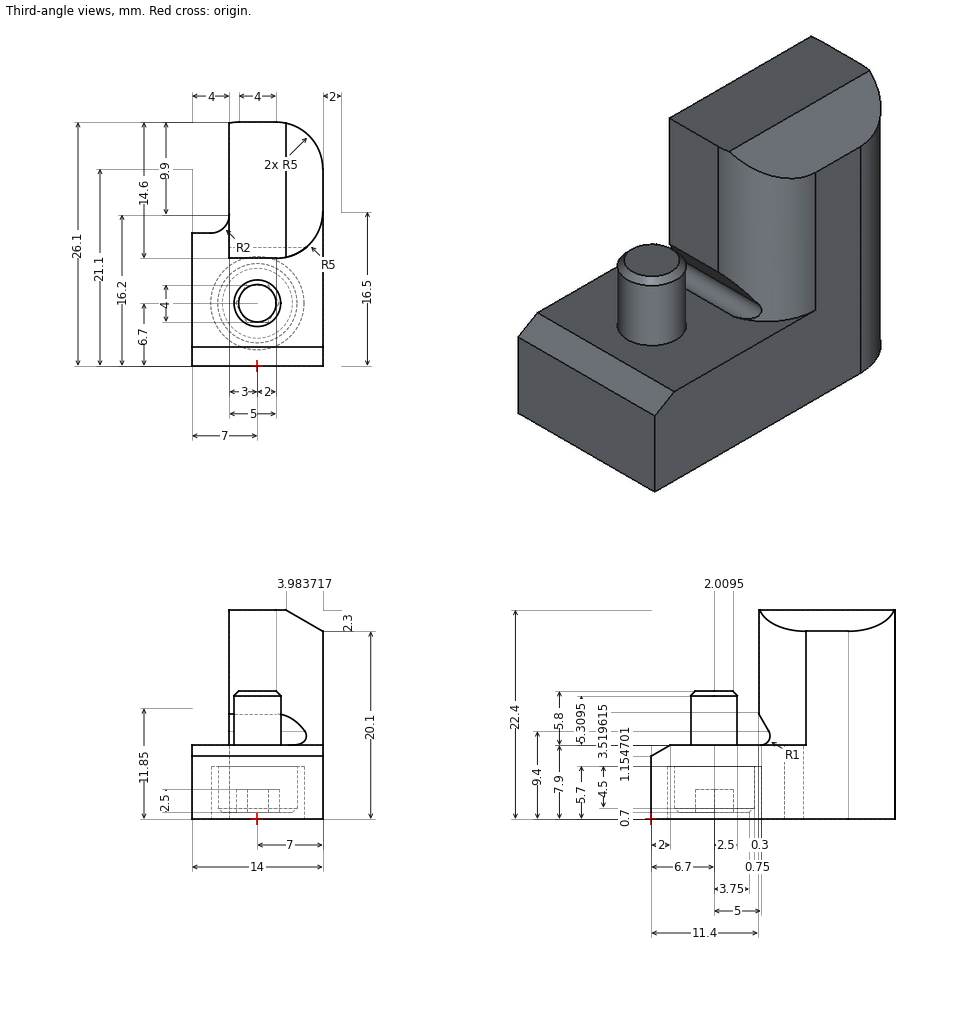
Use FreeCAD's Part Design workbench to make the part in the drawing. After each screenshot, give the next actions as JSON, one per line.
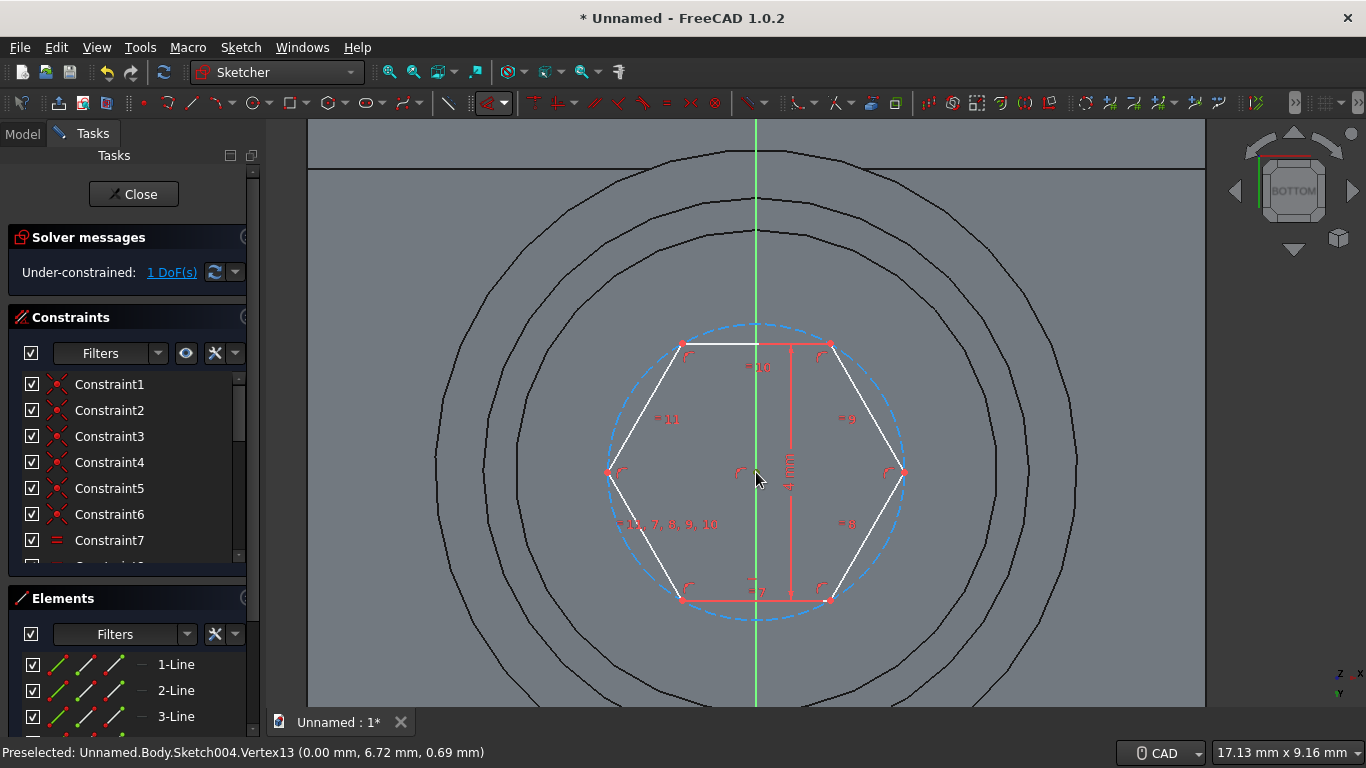
{"action": "left_click", "coordinate": [506, 104]}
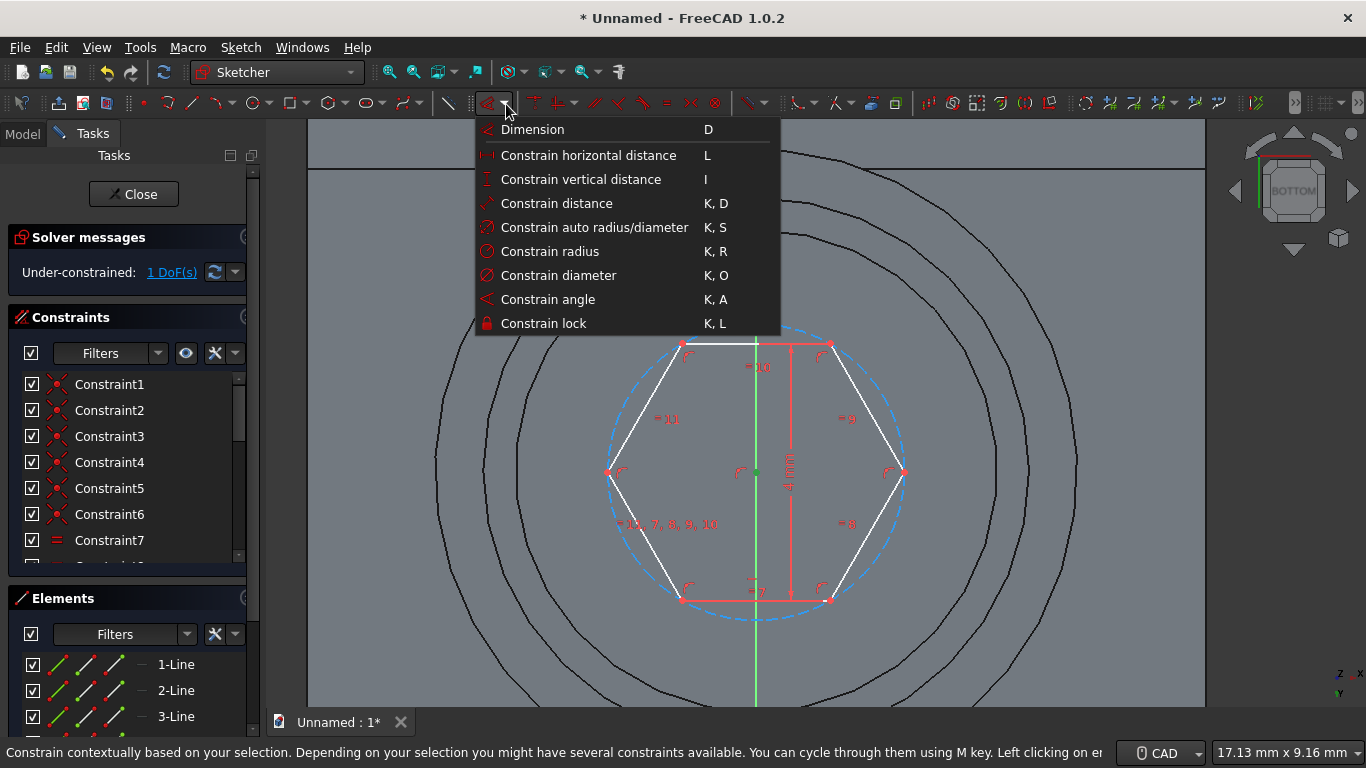
{"action": "left_click", "coordinate": [628, 179]}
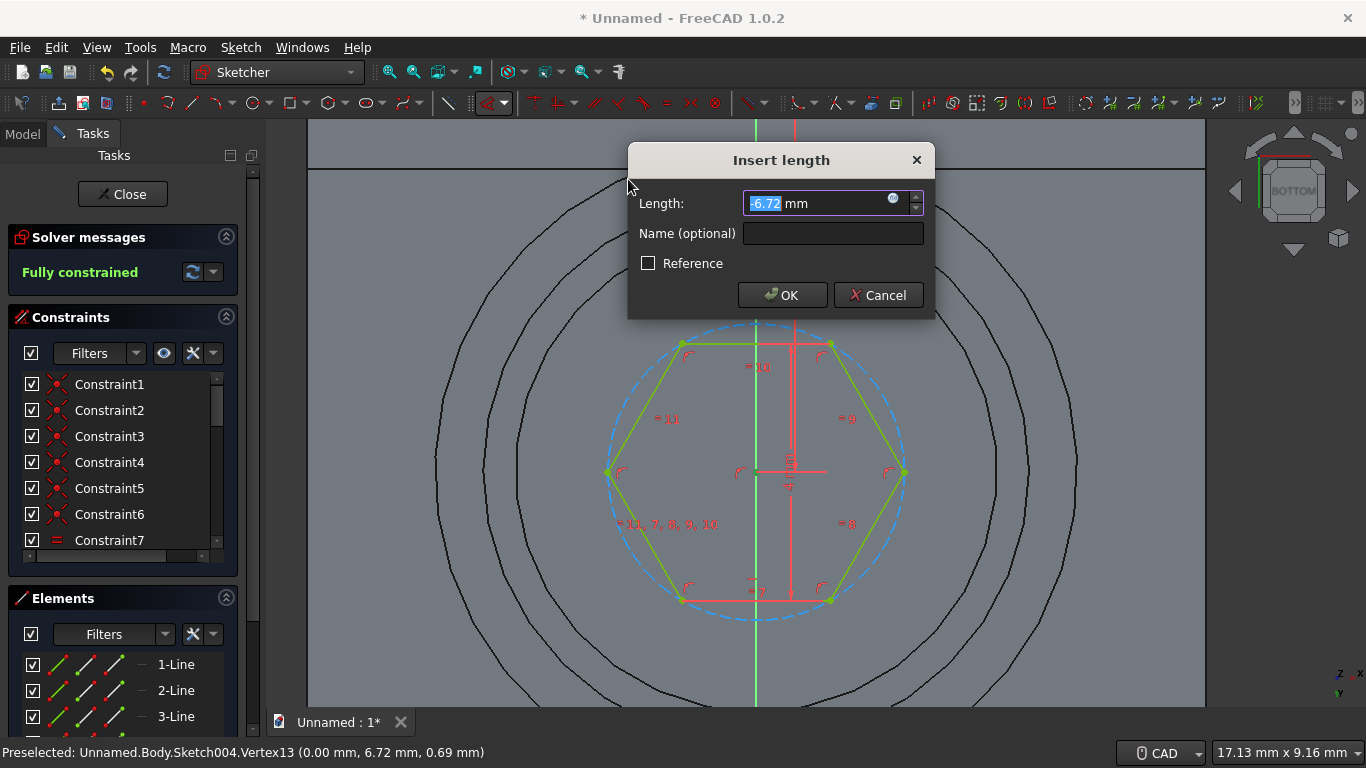
{"action": "type", "text": "-6.7"}
{"action": "key", "text": "Return"}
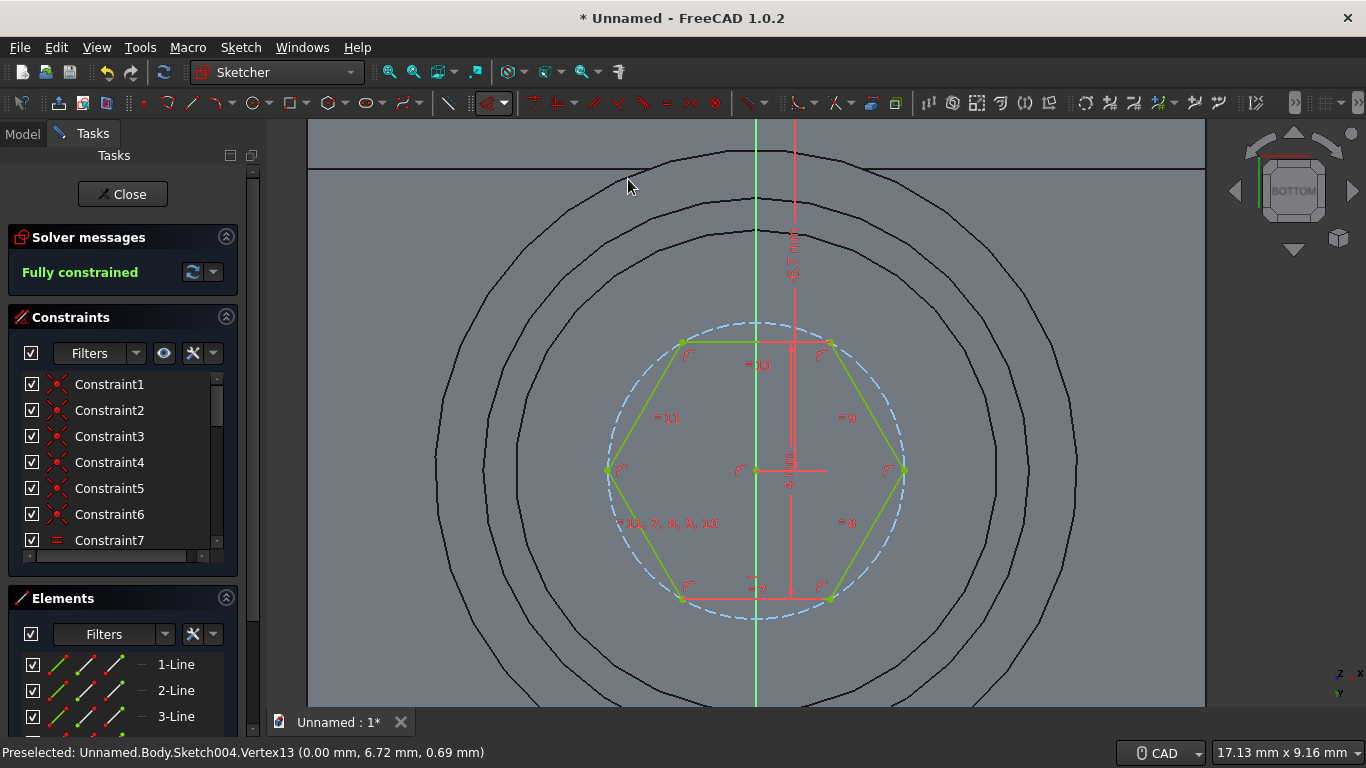
{"action": "left_click", "coordinate": [123, 194]}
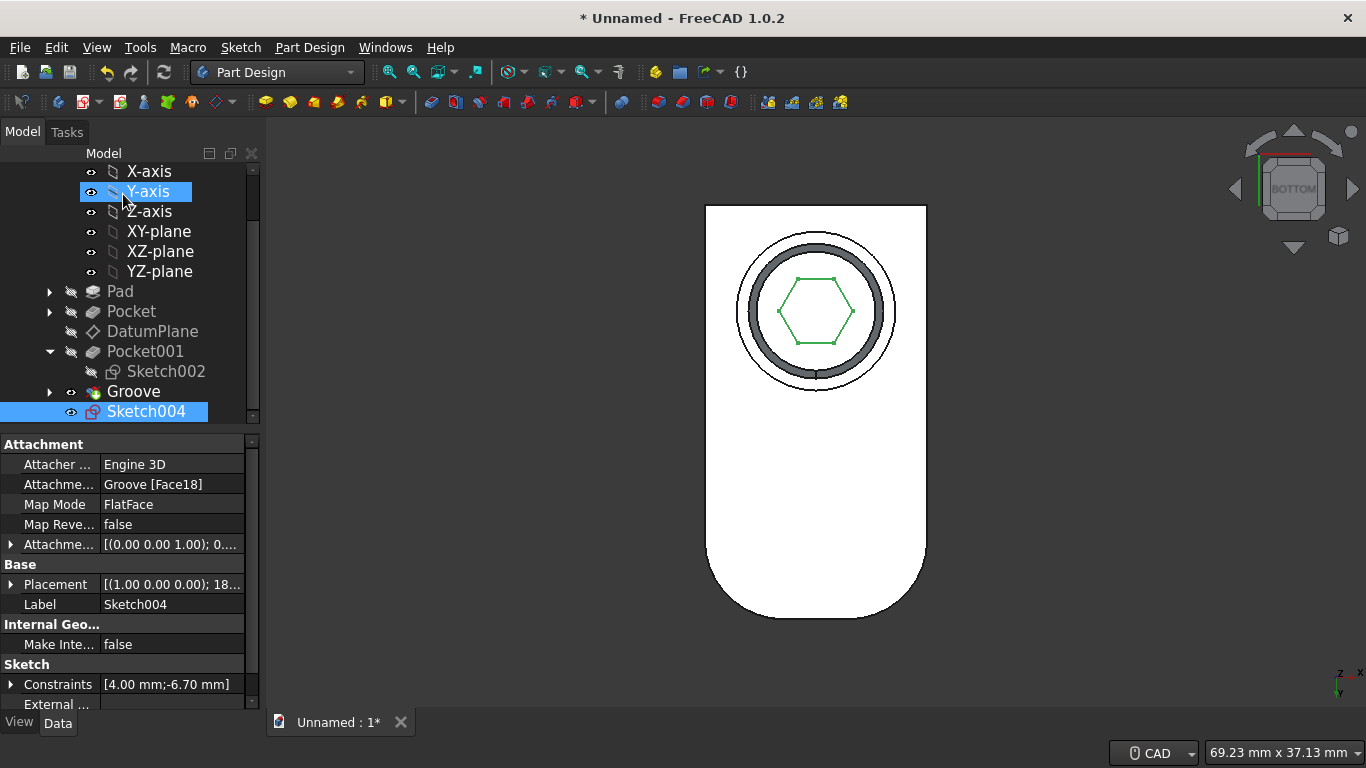
{"action": "left_click", "coordinate": [432, 102]}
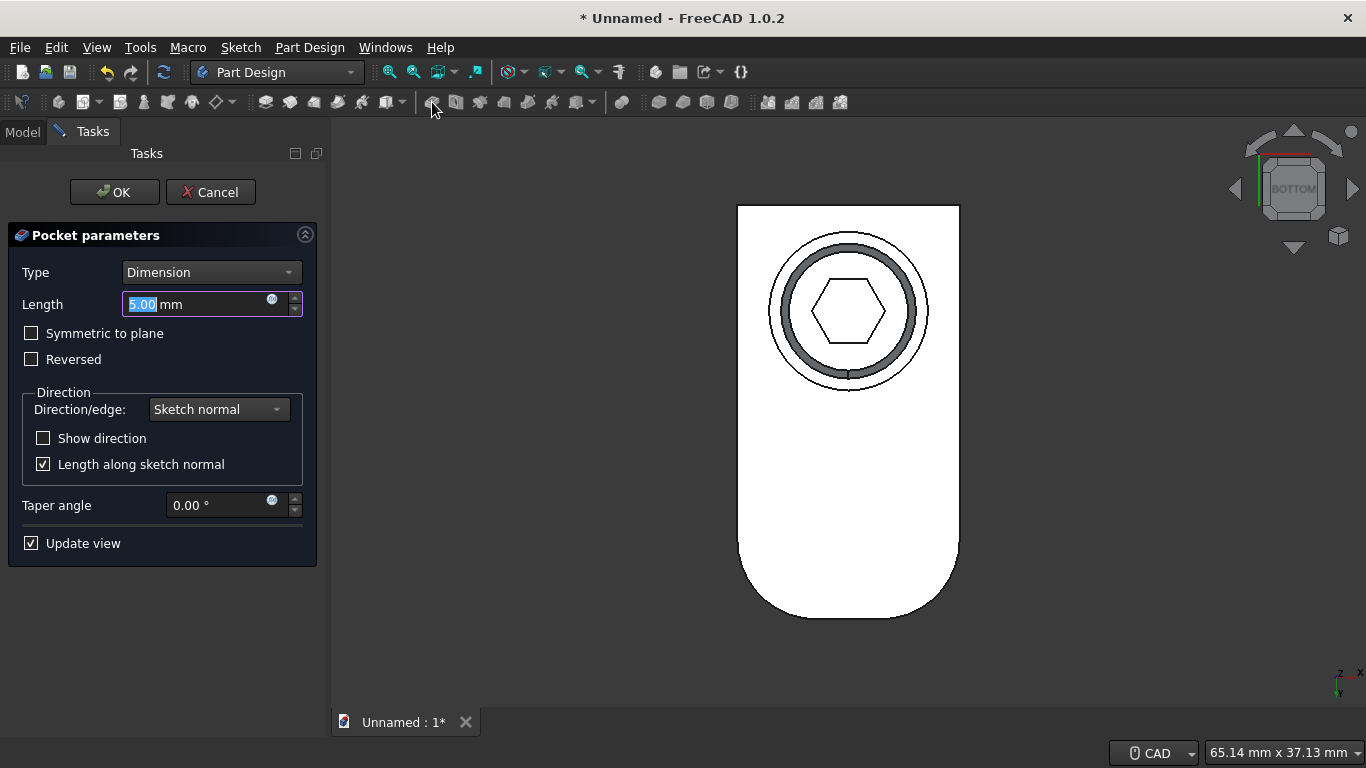
{"action": "type", "text": "2.5"}
{"action": "key", "text": "Tab"}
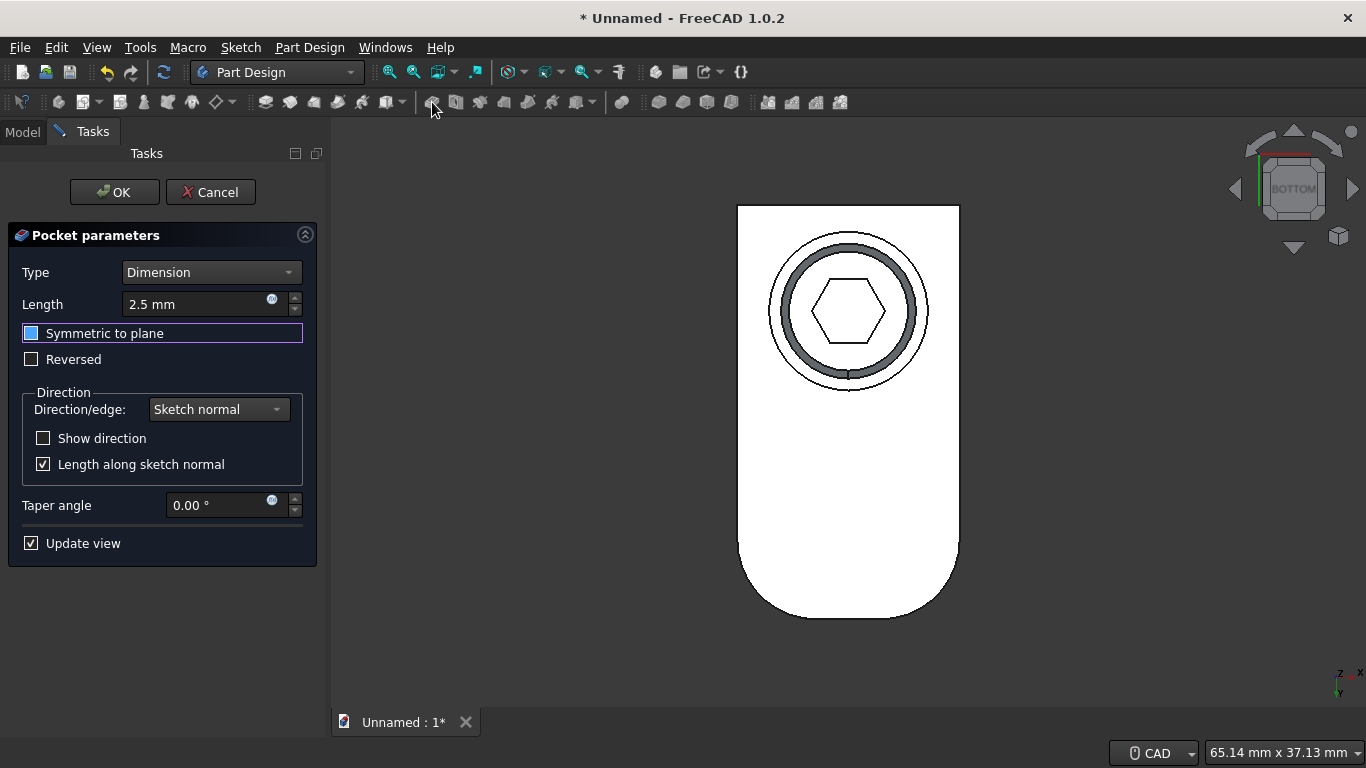
{"action": "left_click", "coordinate": [115, 192]}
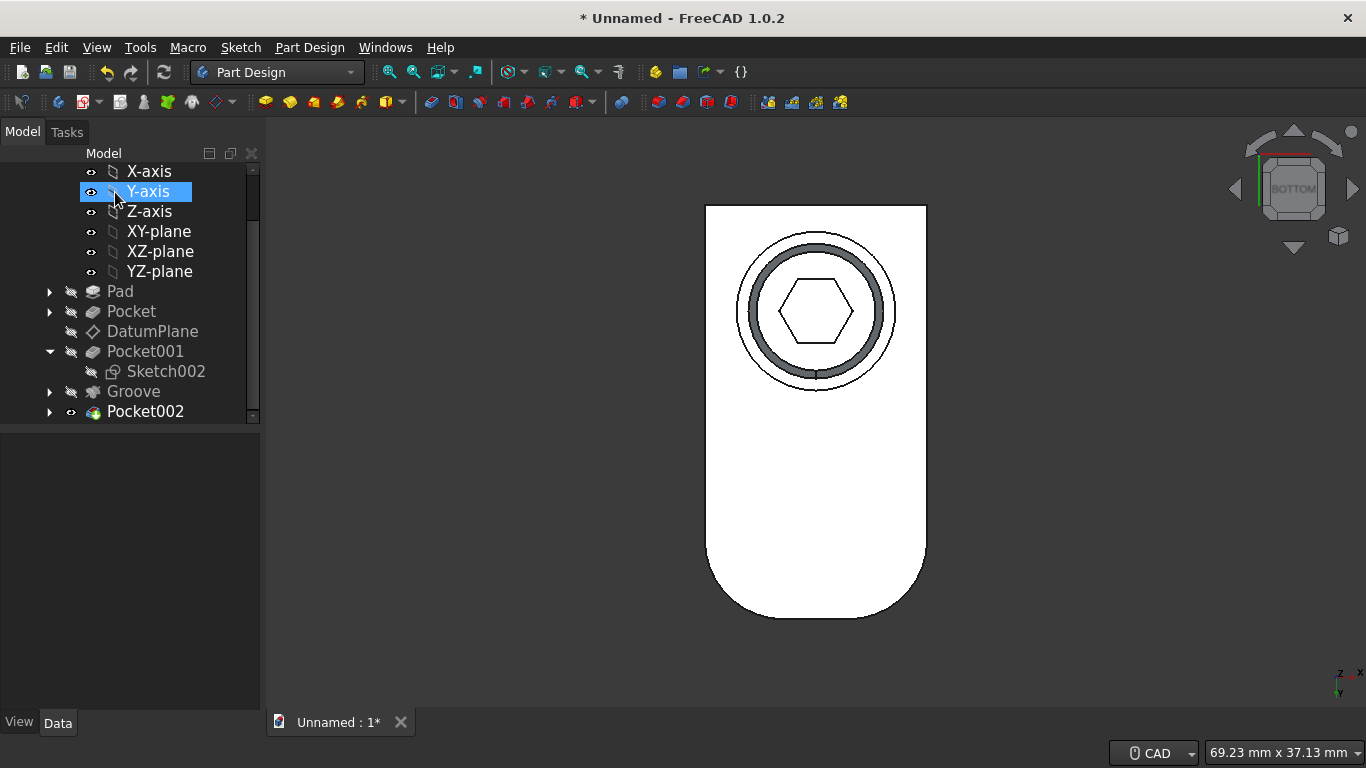
{"action": "scroll", "coordinate": [160, 287], "scroll_direction": "down", "scroll_amount": 3}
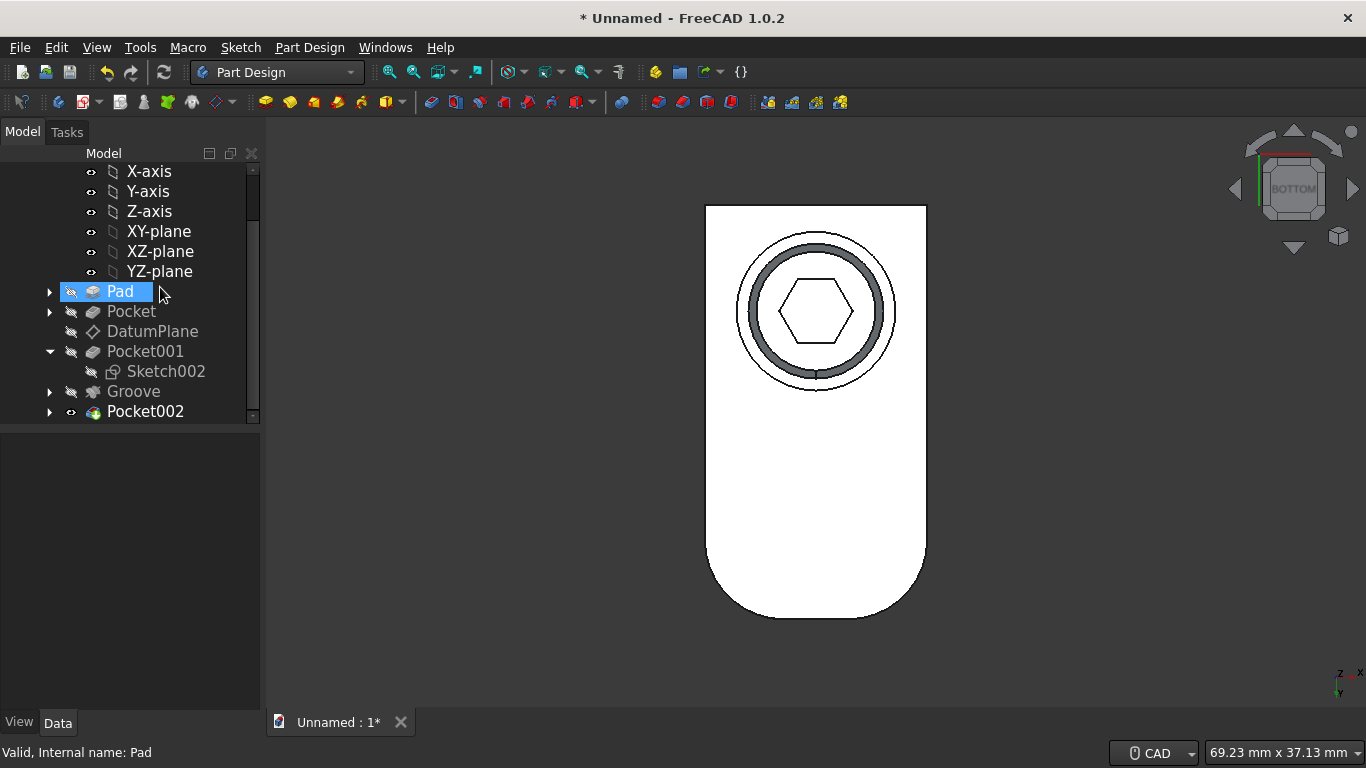
{"action": "scroll", "coordinate": [160, 287], "scroll_direction": "up", "scroll_amount": 15}